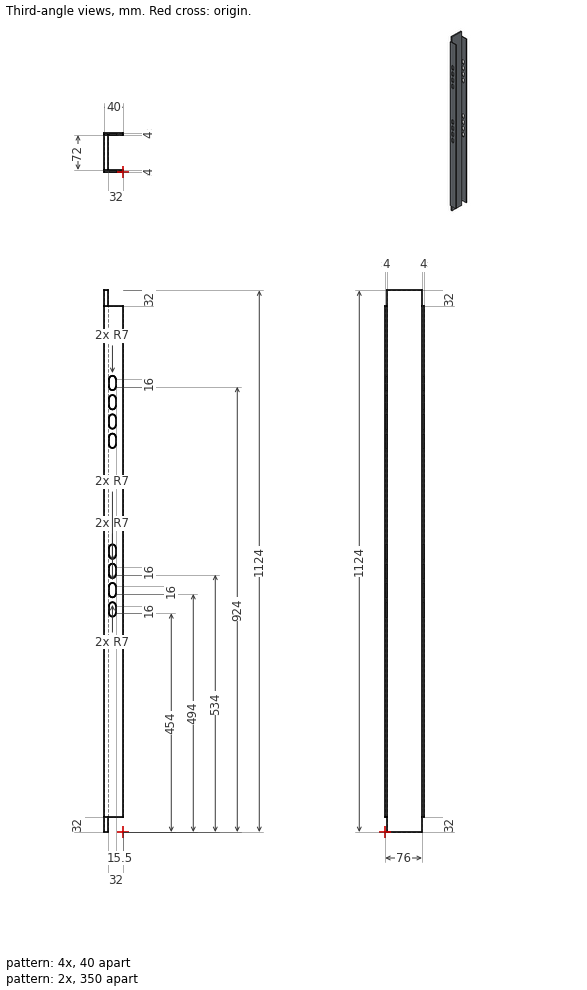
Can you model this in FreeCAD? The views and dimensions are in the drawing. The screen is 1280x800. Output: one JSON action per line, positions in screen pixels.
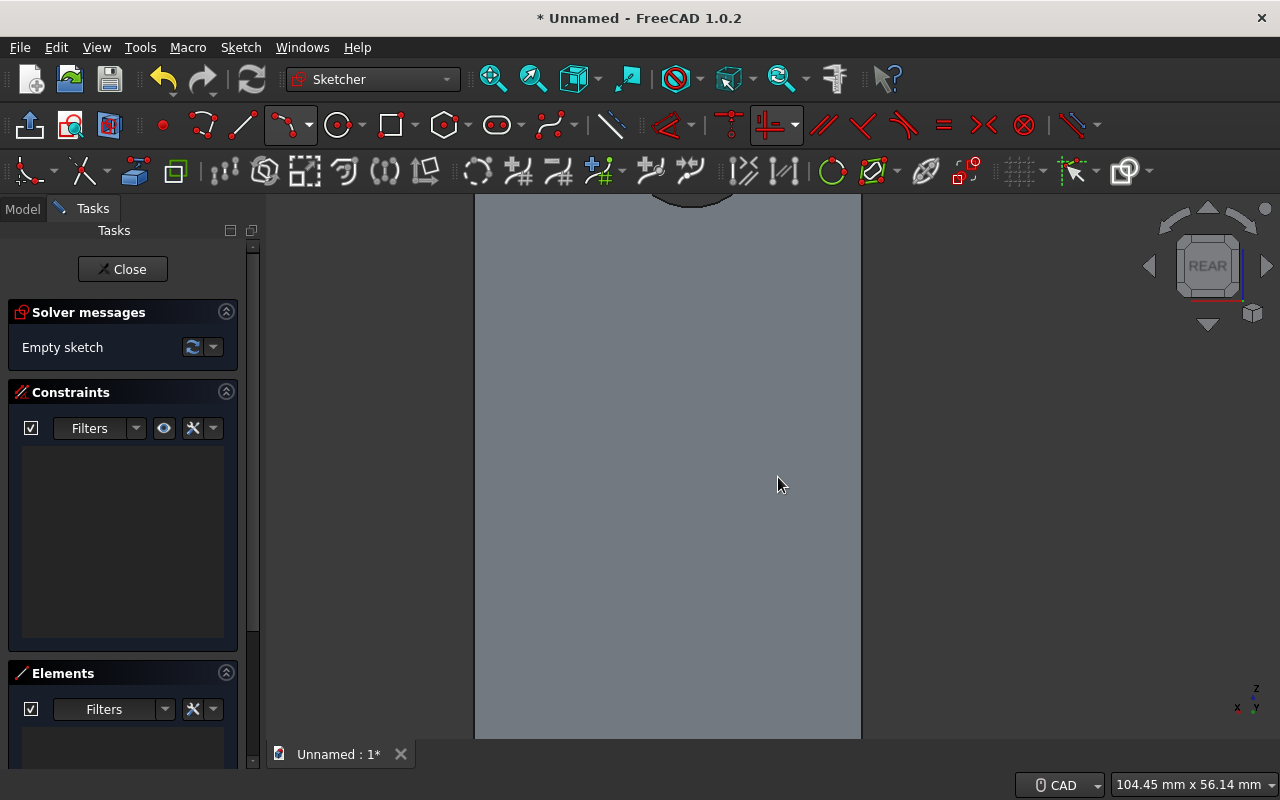
{"action": "key", "text": "g s"}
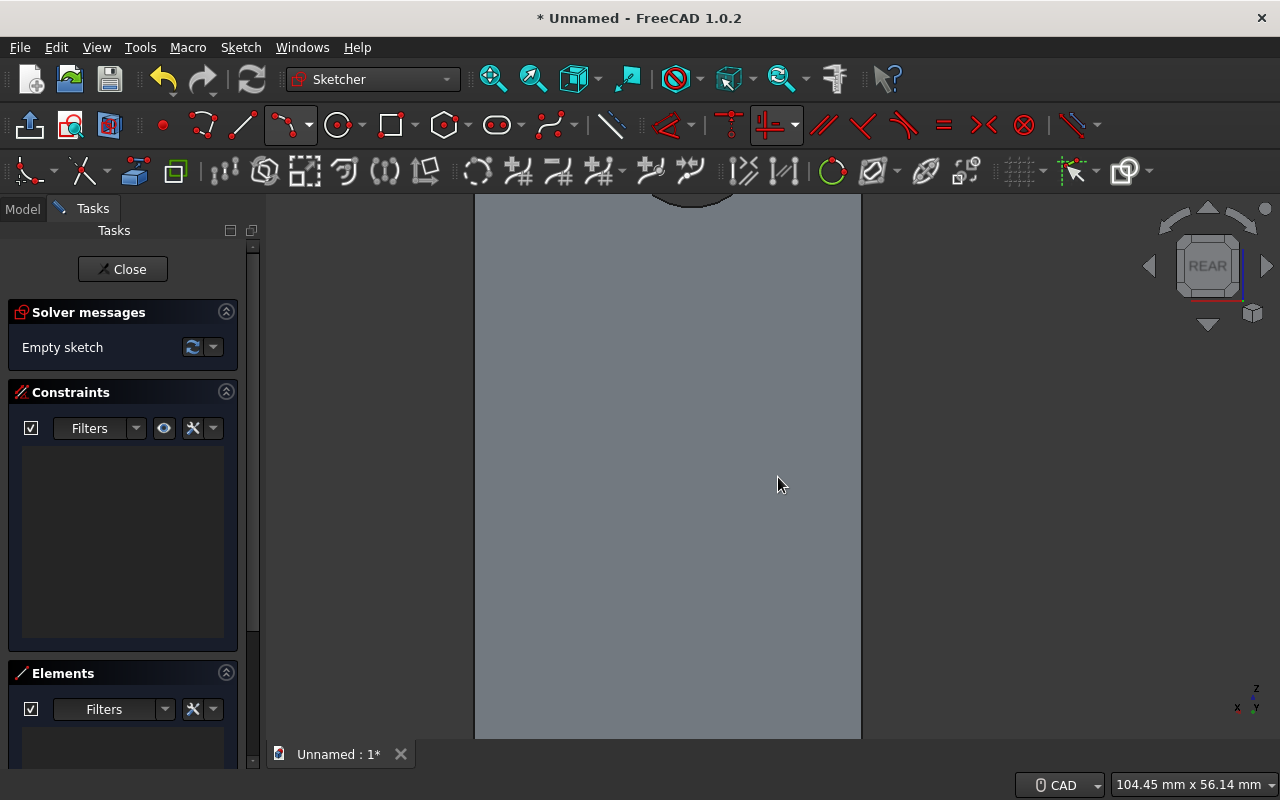
{"action": "left_click", "coordinate": [692, 528]}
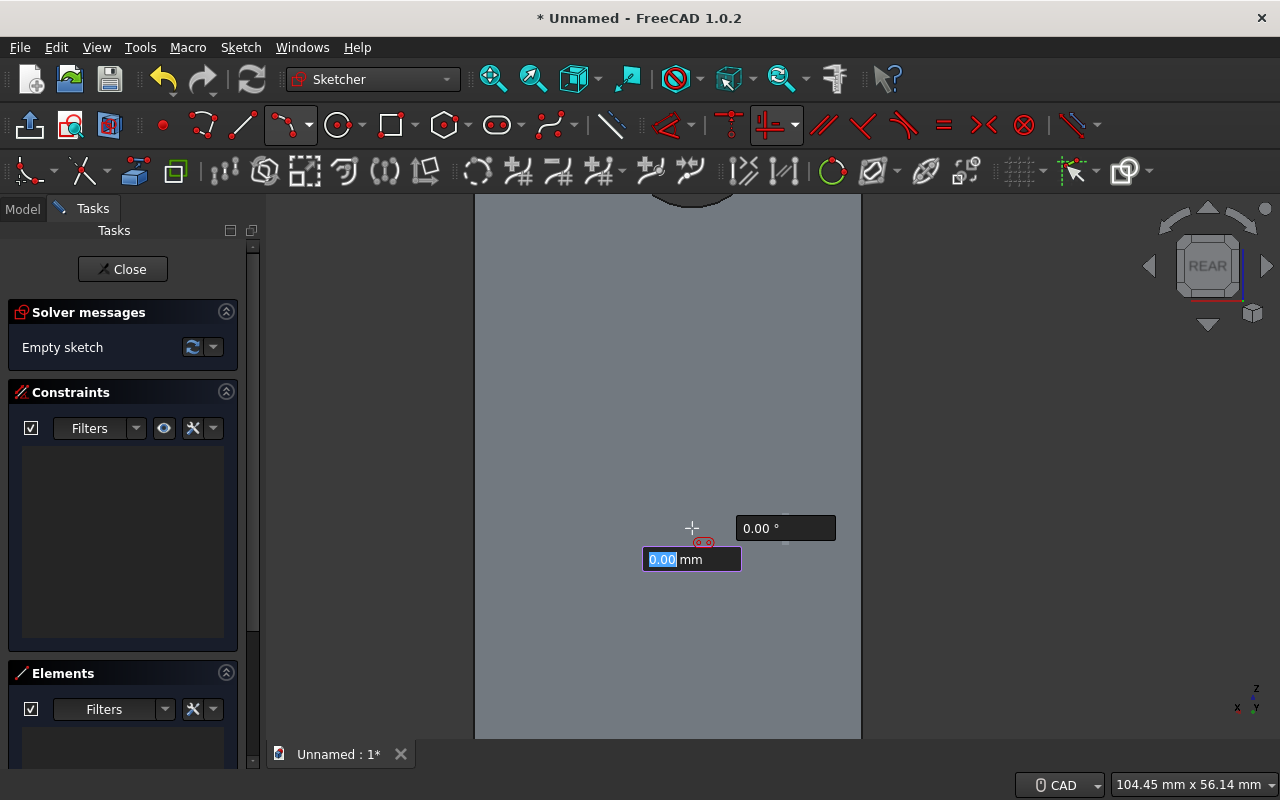
{"action": "left_click", "coordinate": [692, 373]}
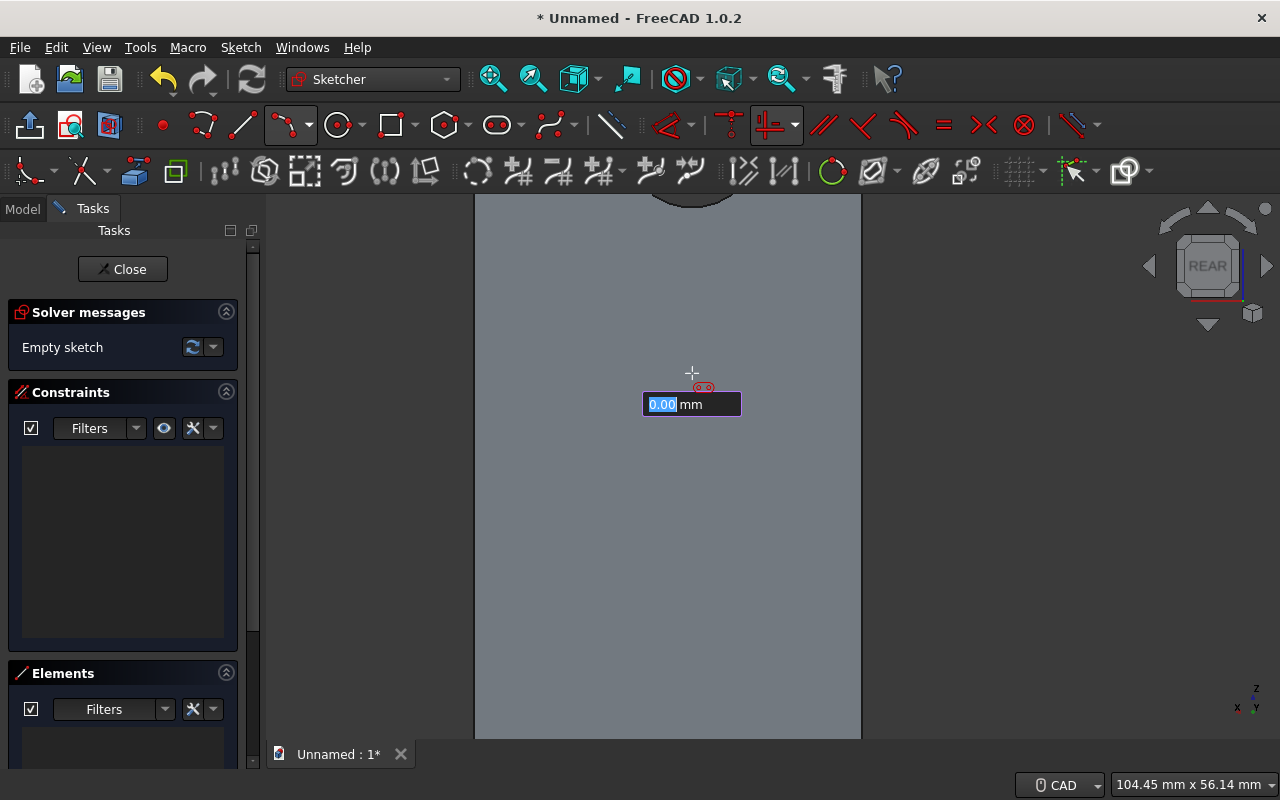
{"action": "left_click", "coordinate": [760, 450]}
{"action": "key", "text": "Escape"}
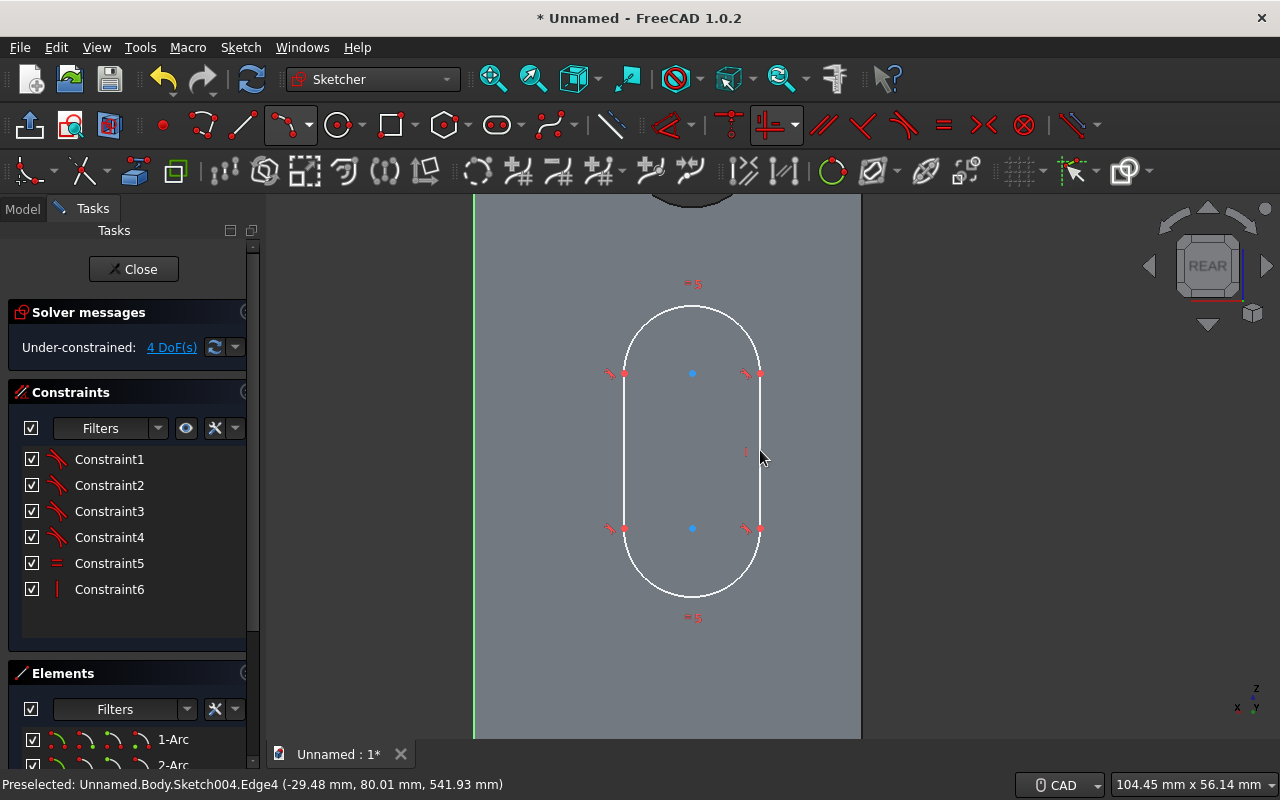
{"action": "left_click", "coordinate": [666, 126]}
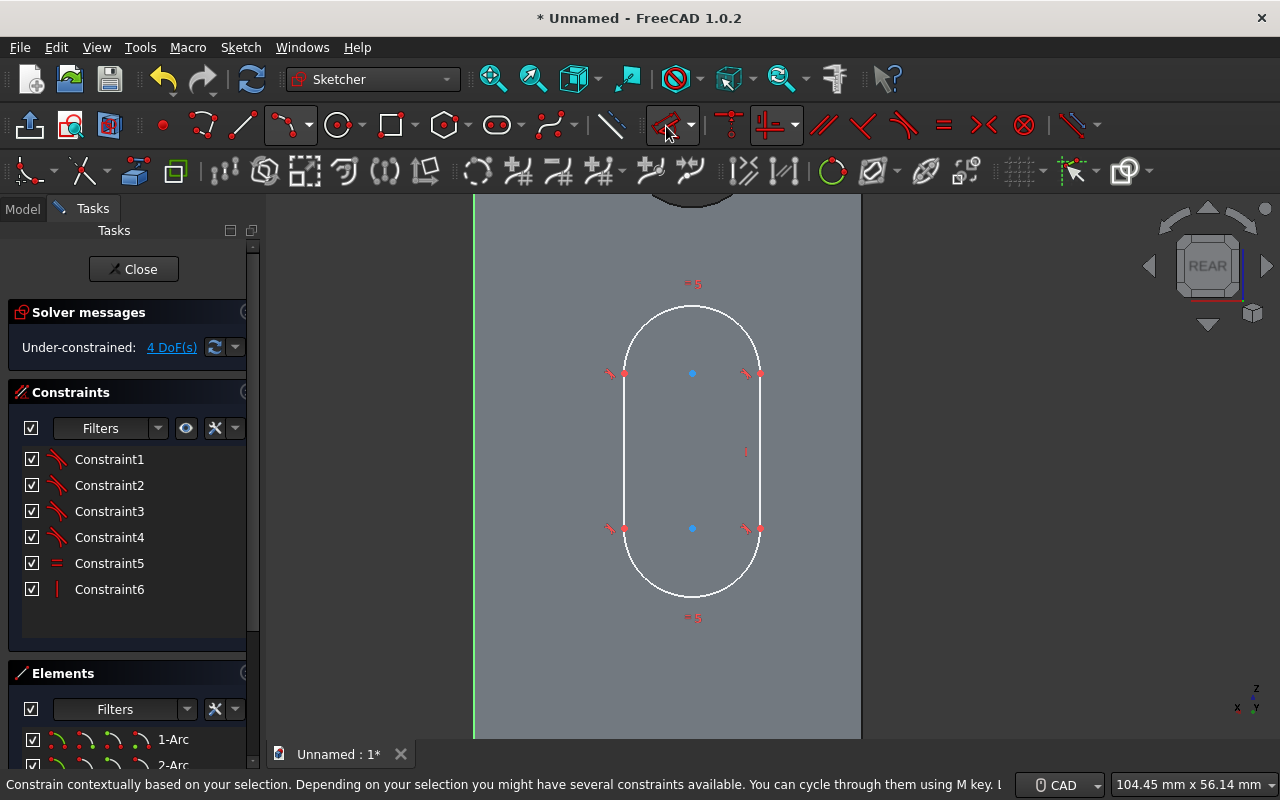
{"action": "left_click", "coordinate": [652, 584]}
{"action": "left_click", "coordinate": [633, 610]}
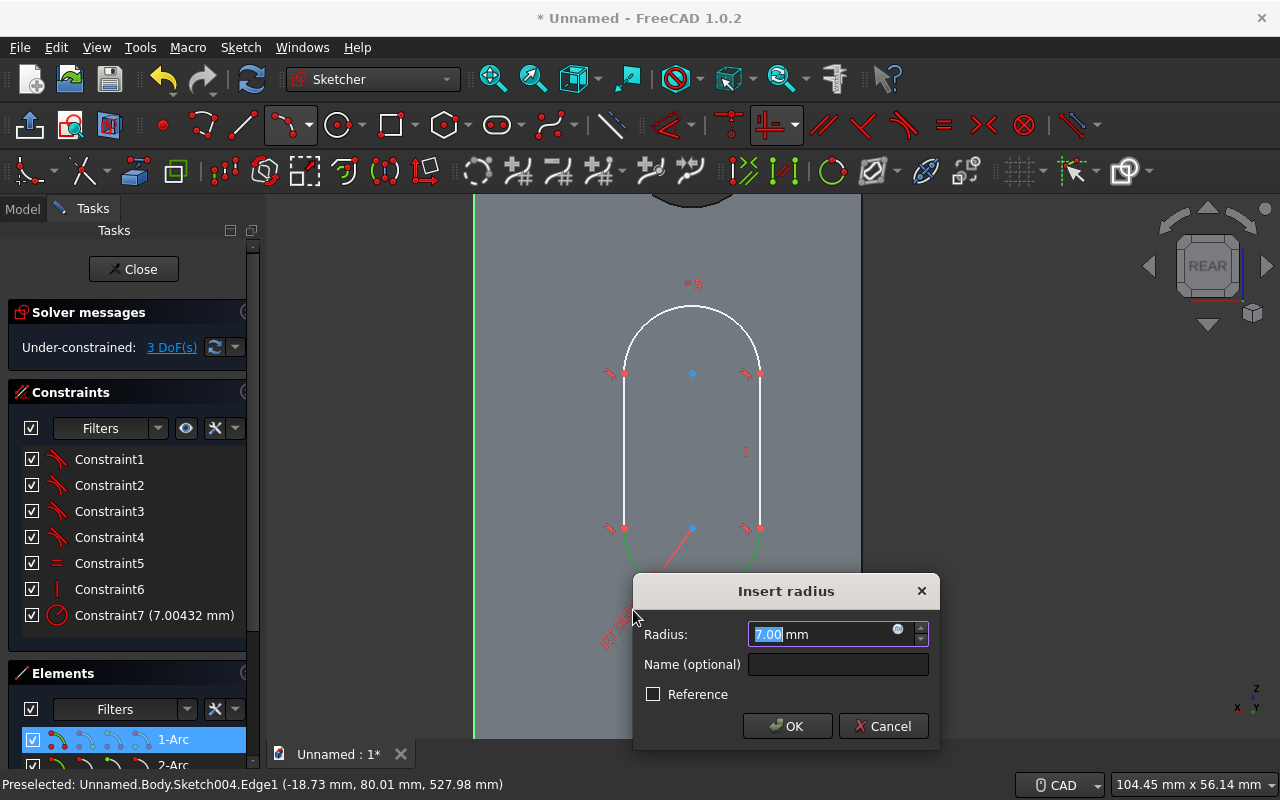
{"action": "type", "text": "7"}
{"action": "key", "text": "Return"}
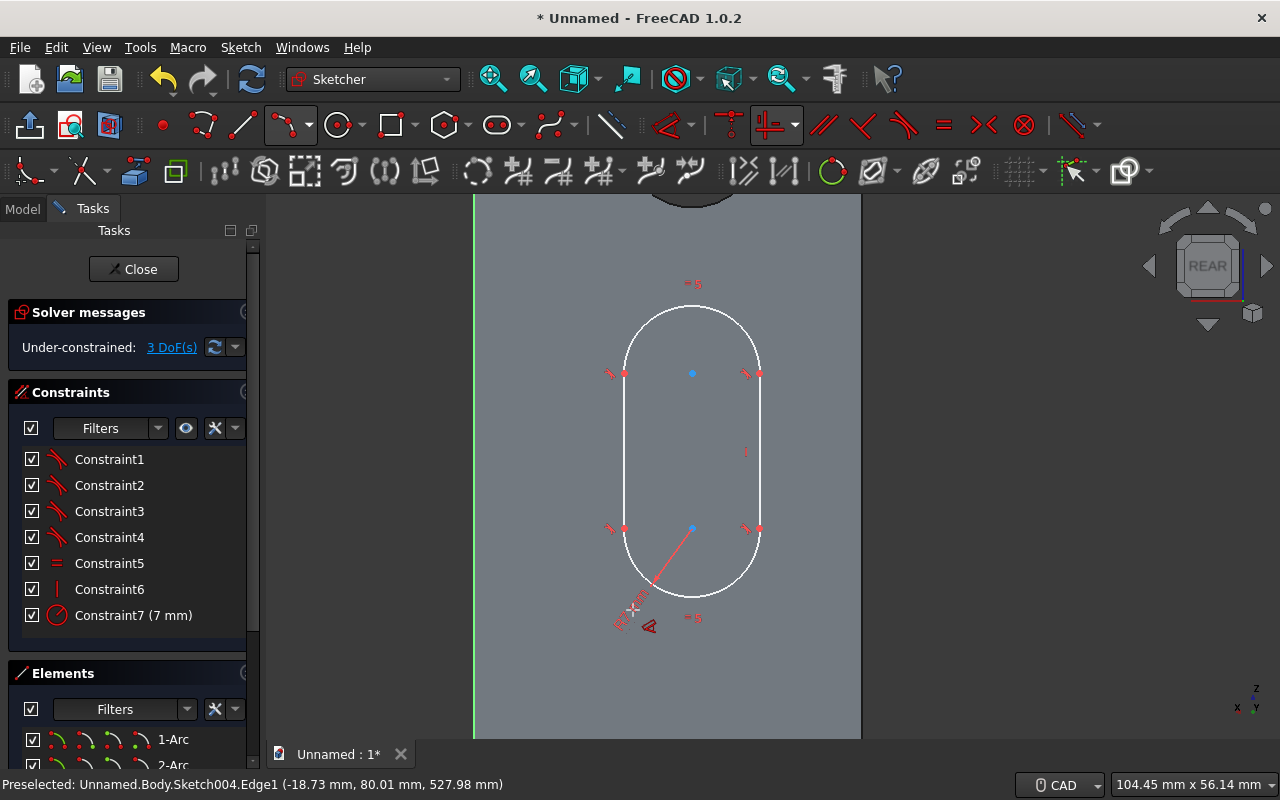
{"action": "left_click", "coordinate": [624, 483]}
{"action": "left_click", "coordinate": [590, 451]}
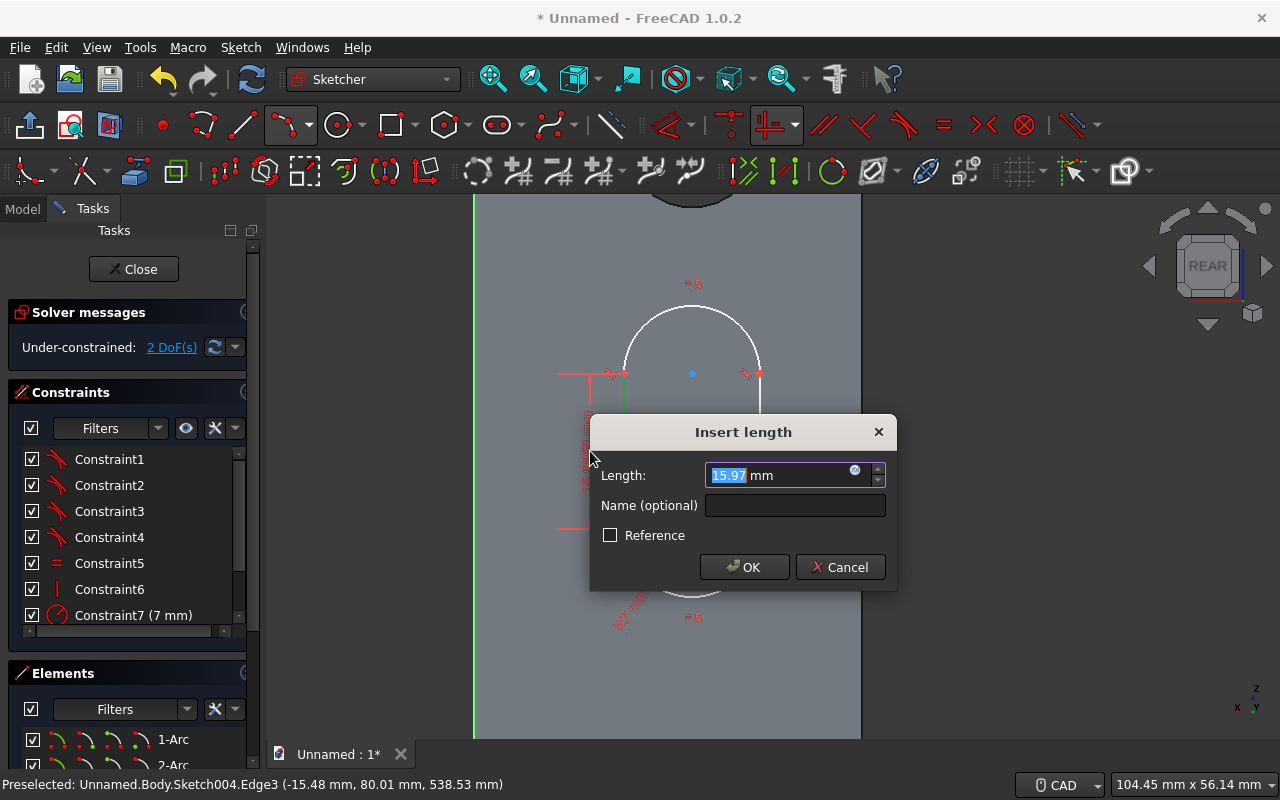
{"action": "type", "text": "16"}
{"action": "key", "text": "Return"}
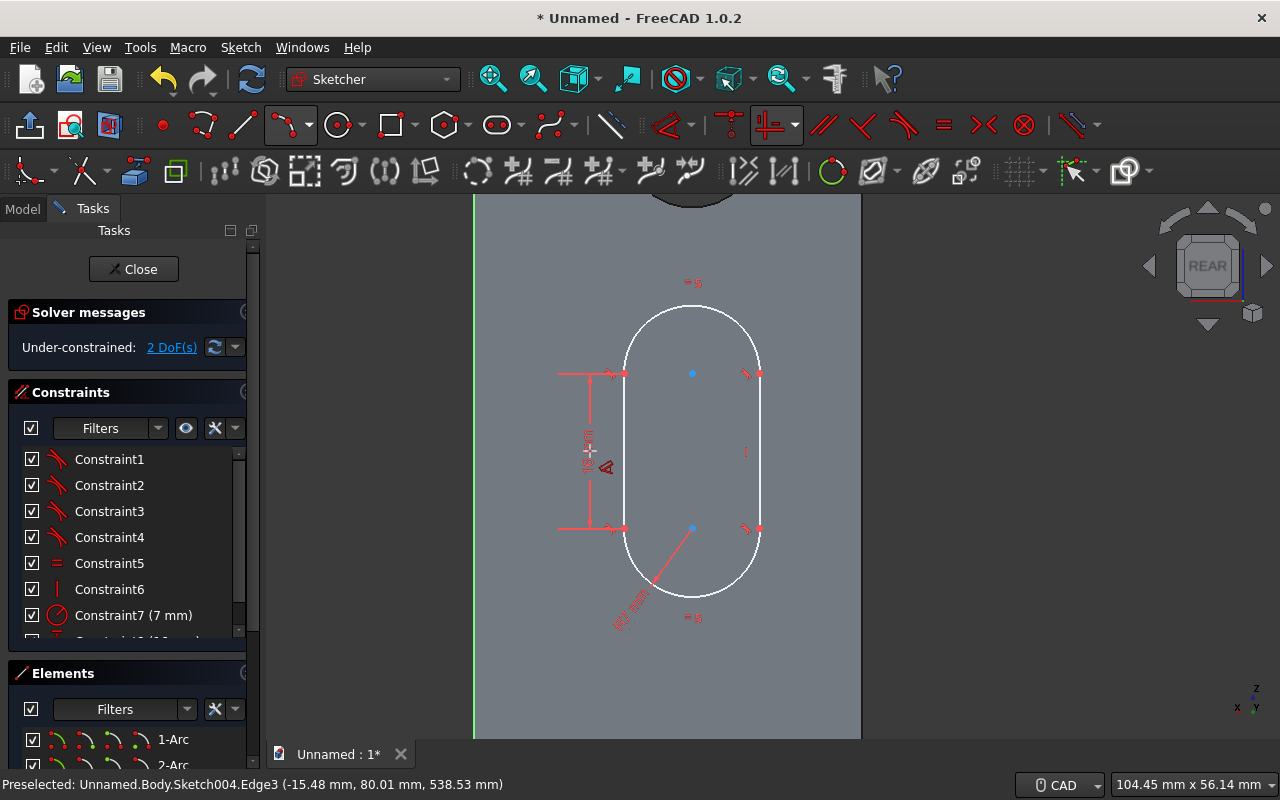
{"action": "left_click", "coordinate": [624, 529]}
{"action": "left_click", "coordinate": [440, 620]}